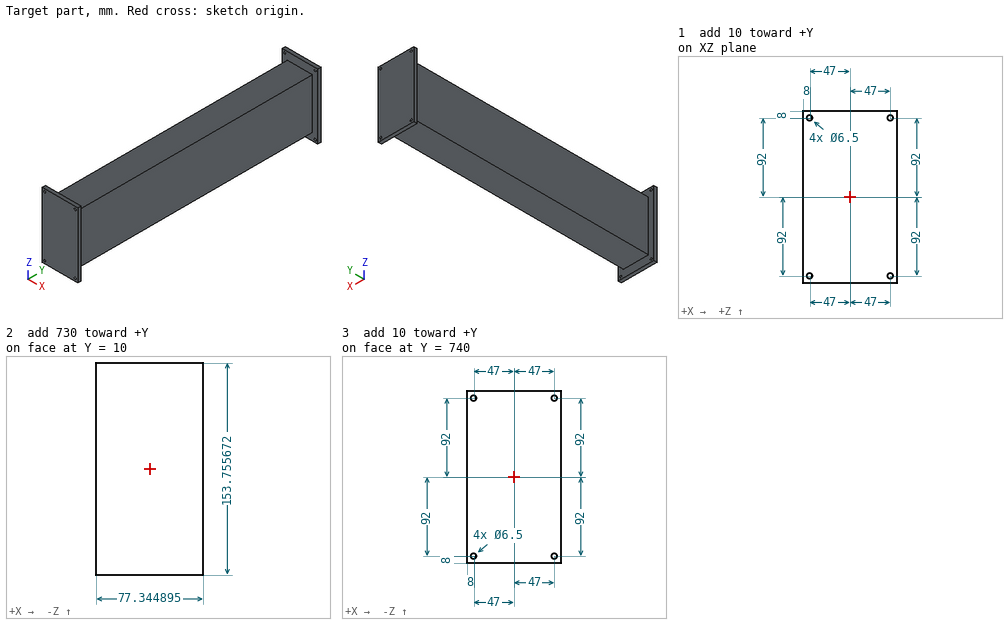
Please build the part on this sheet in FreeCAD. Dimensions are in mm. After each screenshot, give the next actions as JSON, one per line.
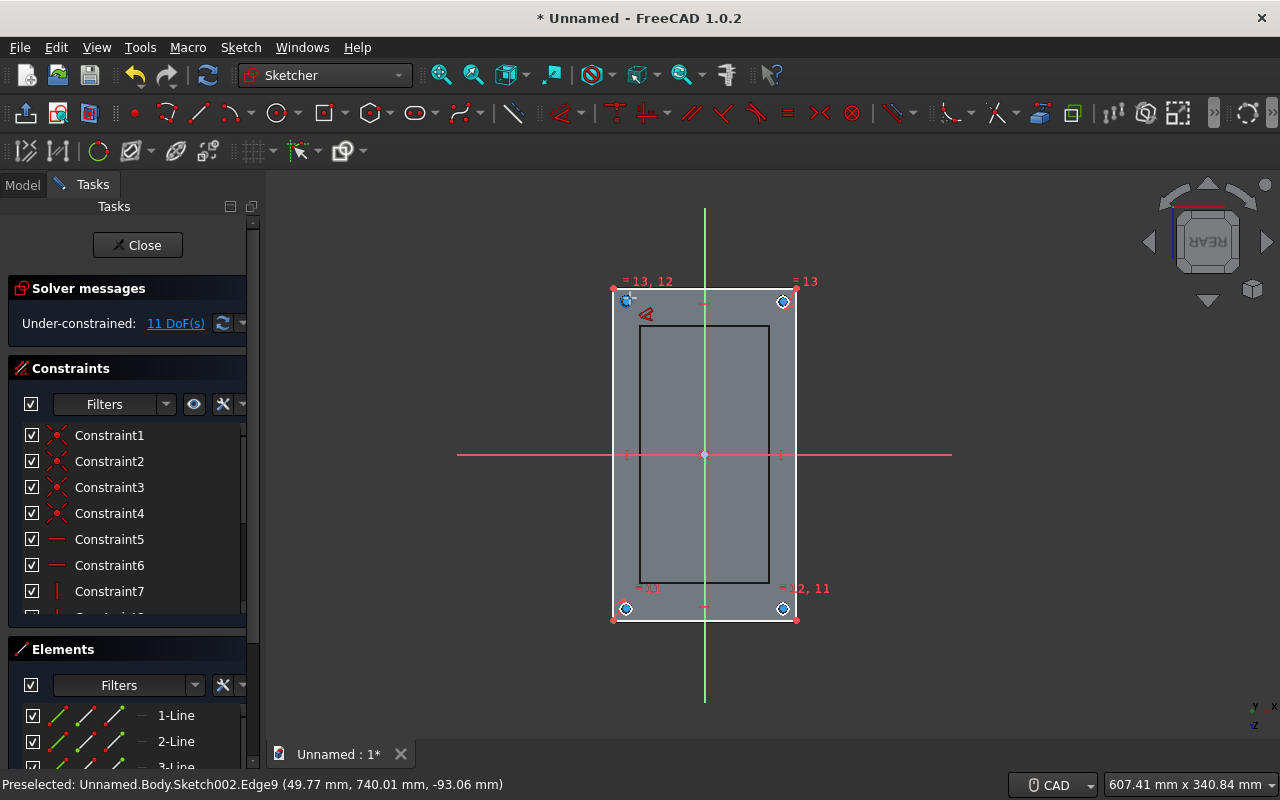
{"action": "scroll", "coordinate": [630, 605], "scroll_direction": "up", "scroll_amount": 7}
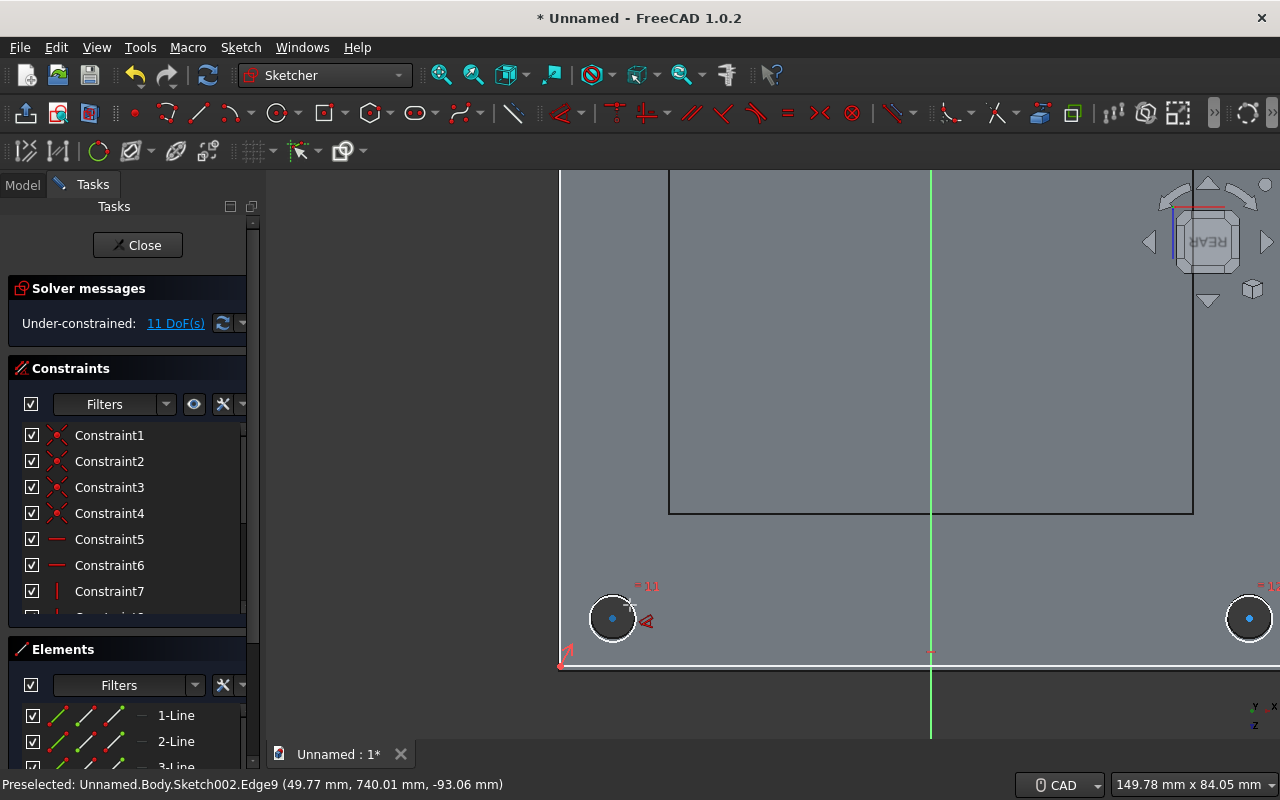
{"action": "left_click", "coordinate": [629, 603]}
{"action": "left_click", "coordinate": [652, 581]}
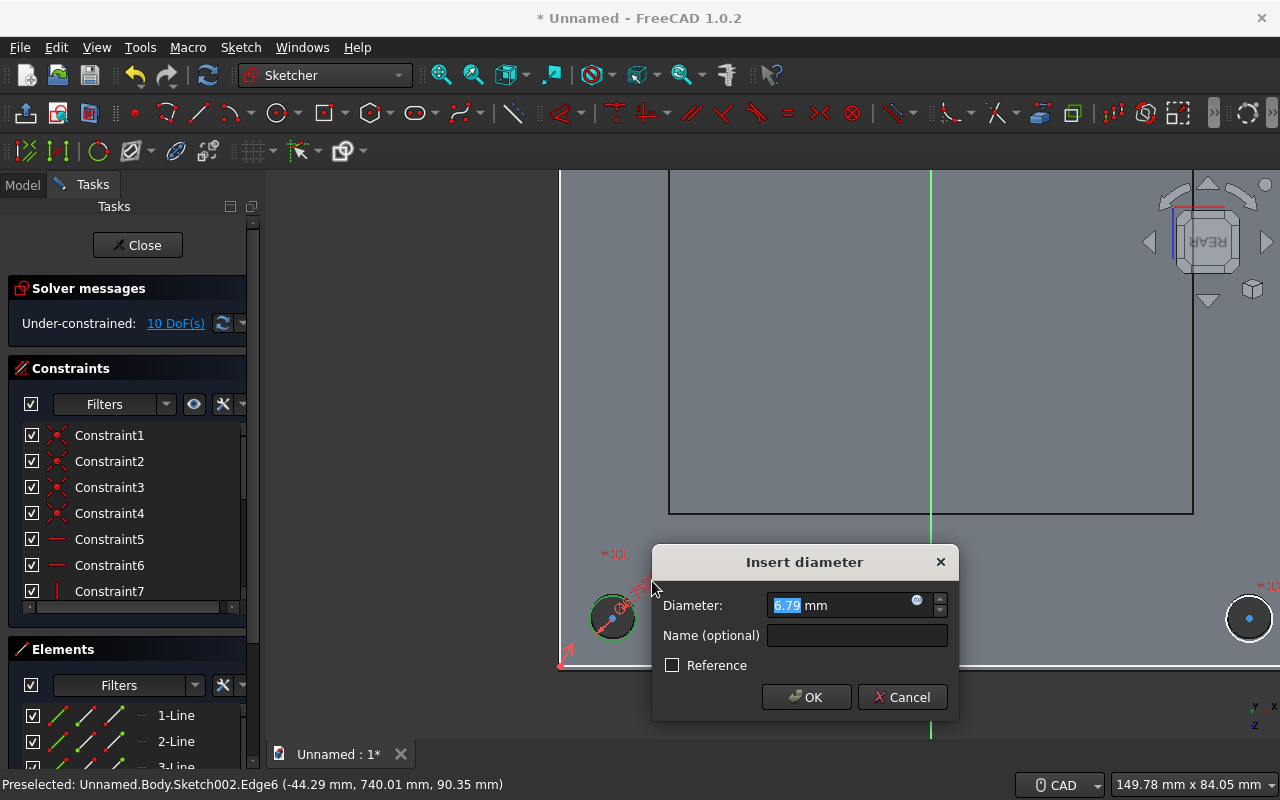
{"action": "type", "text": "6.5"}
{"action": "key", "text": "Return"}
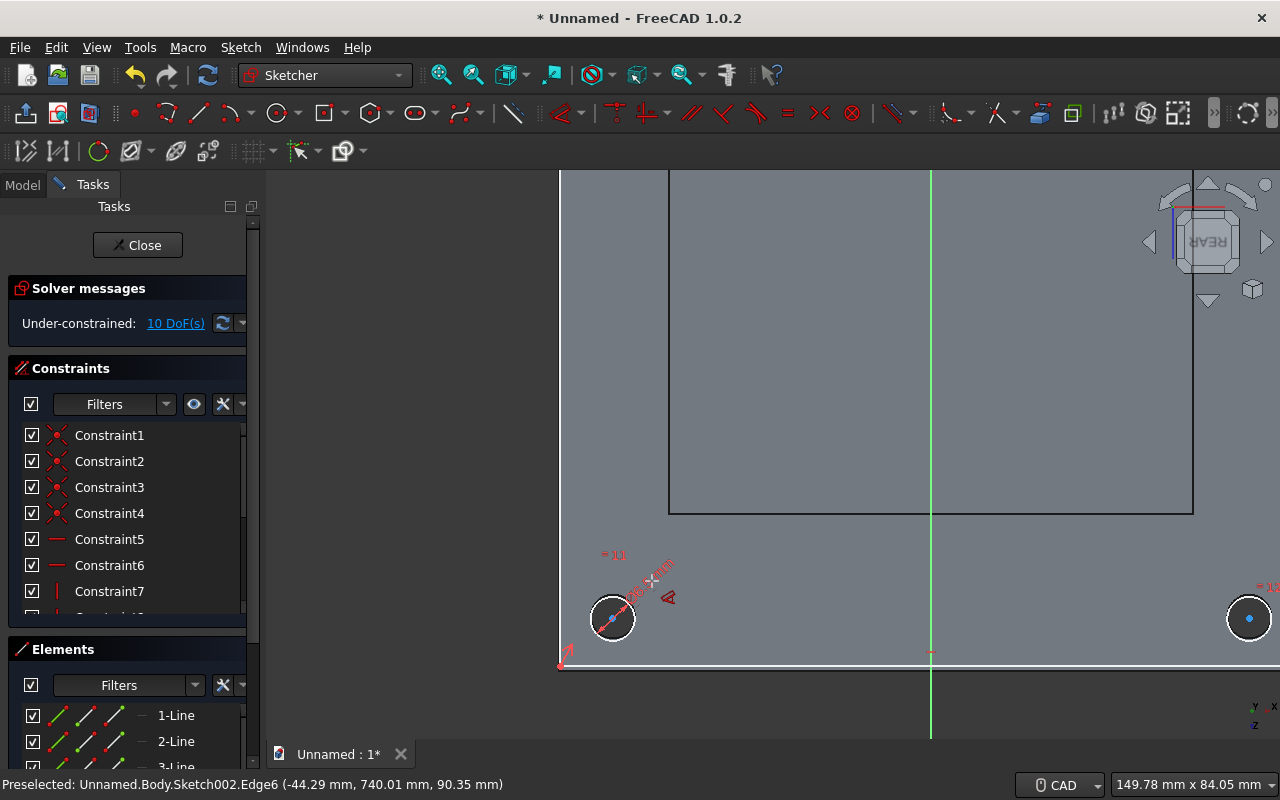
{"action": "scroll", "coordinate": [630, 605], "scroll_direction": "down", "scroll_amount": 7}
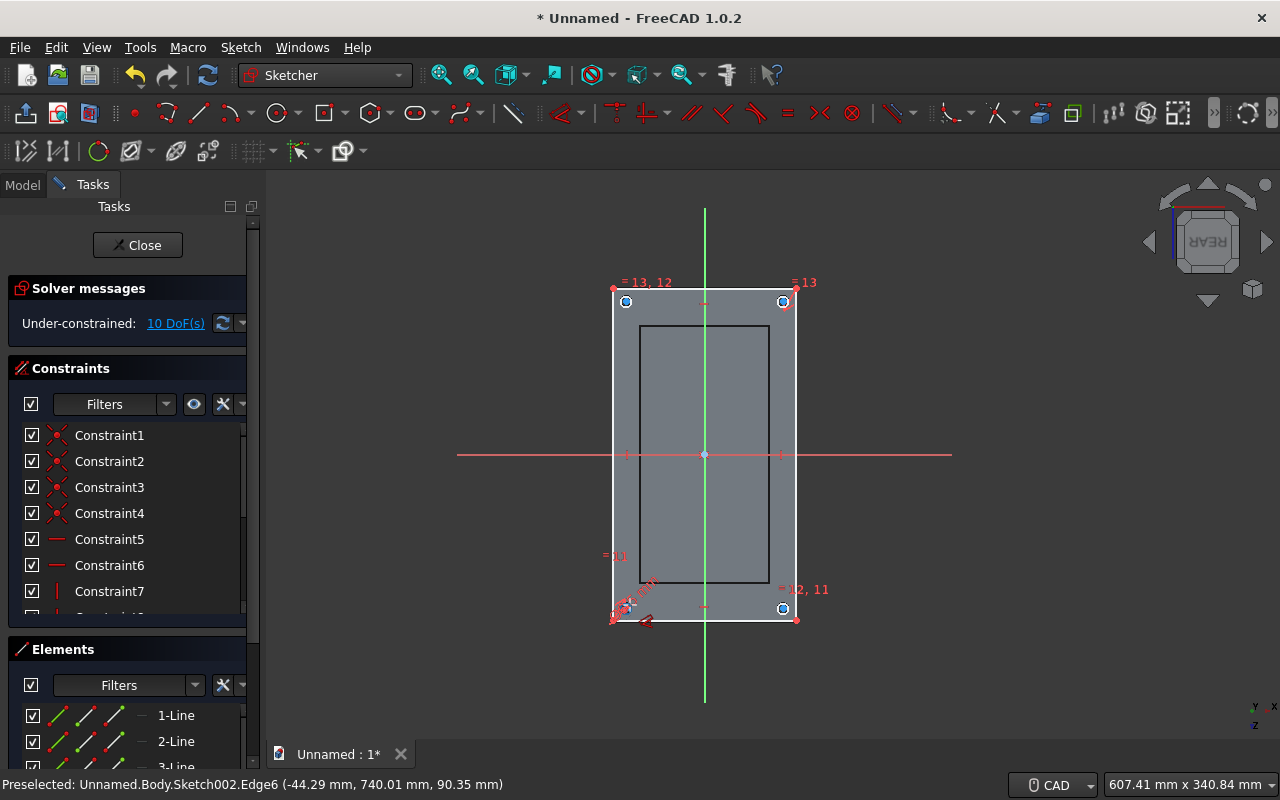
{"action": "left_click", "coordinate": [626, 609]}
{"action": "left_click", "coordinate": [665, 643]}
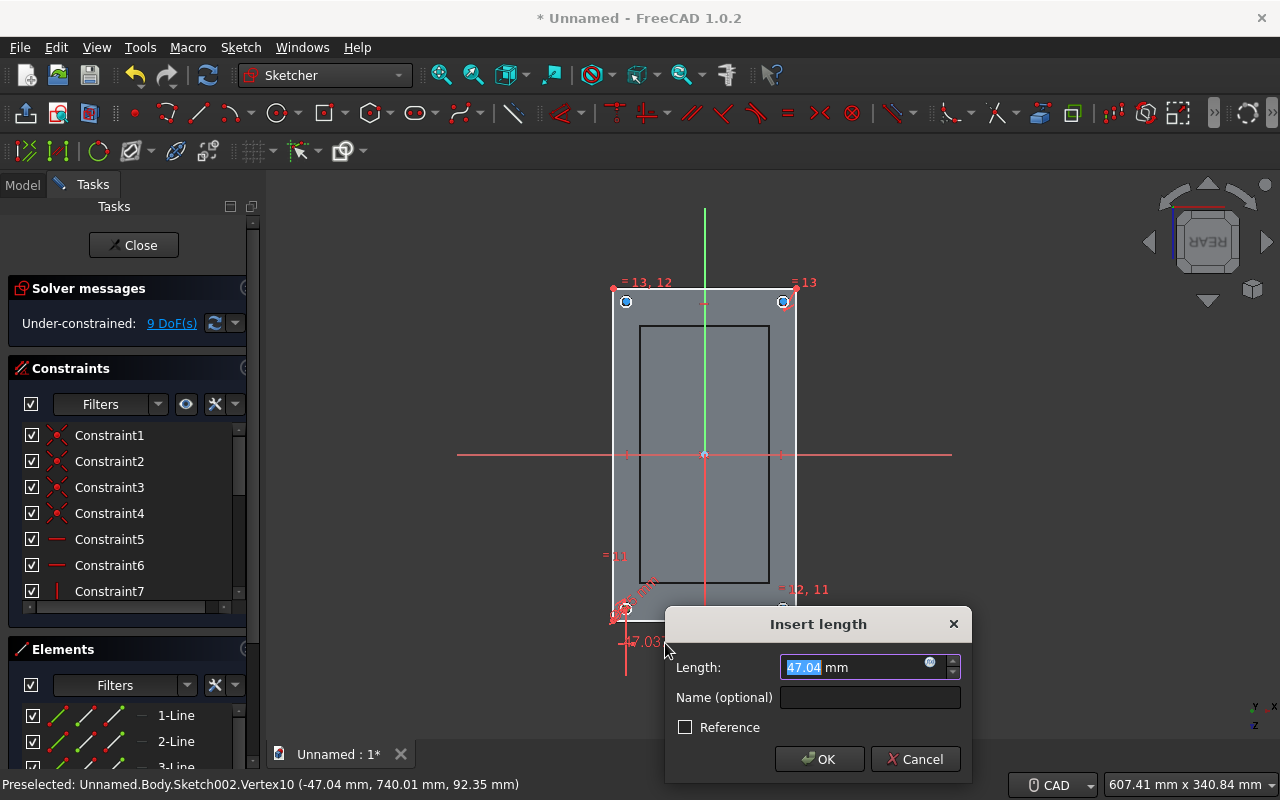
{"action": "type", "text": "47"}
{"action": "key", "text": "Return"}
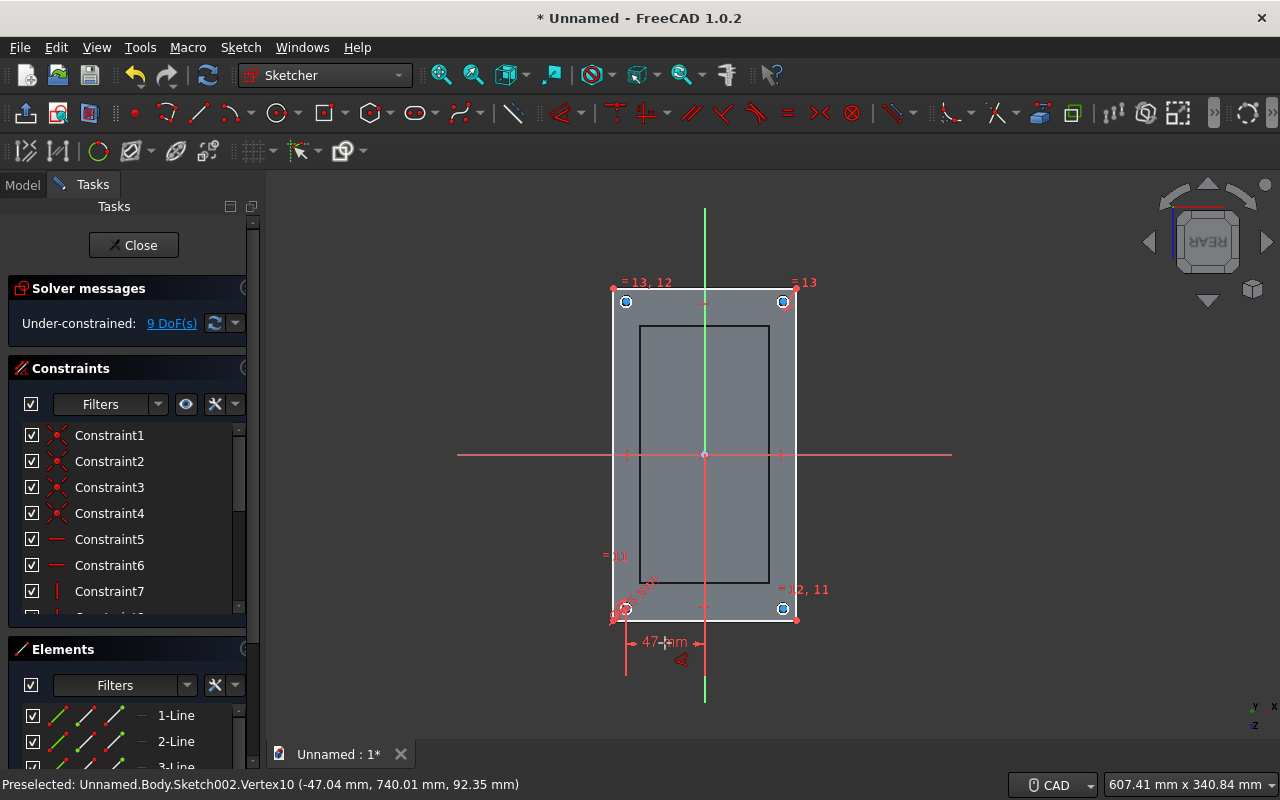
{"action": "left_click", "coordinate": [626, 609]}
{"action": "left_click", "coordinate": [592, 532]}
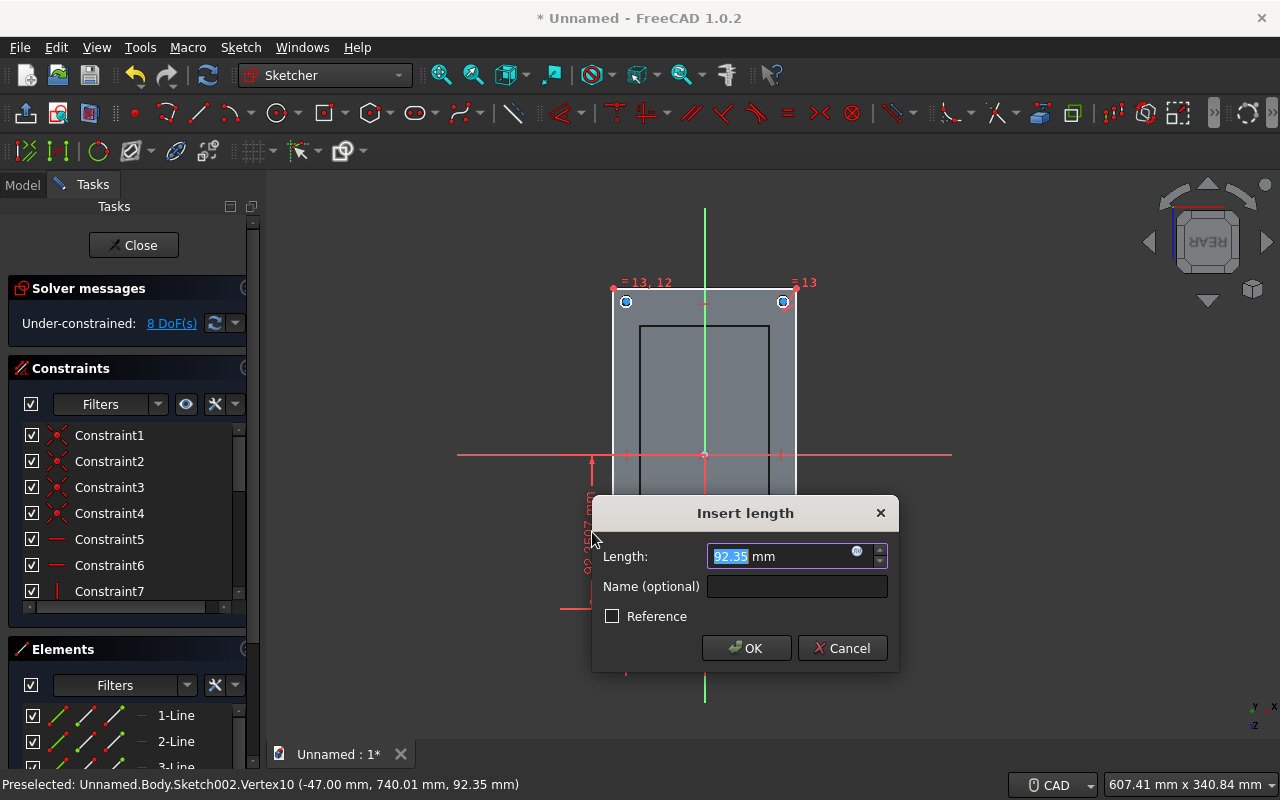
{"action": "type", "text": "92"}
{"action": "key", "text": "Return"}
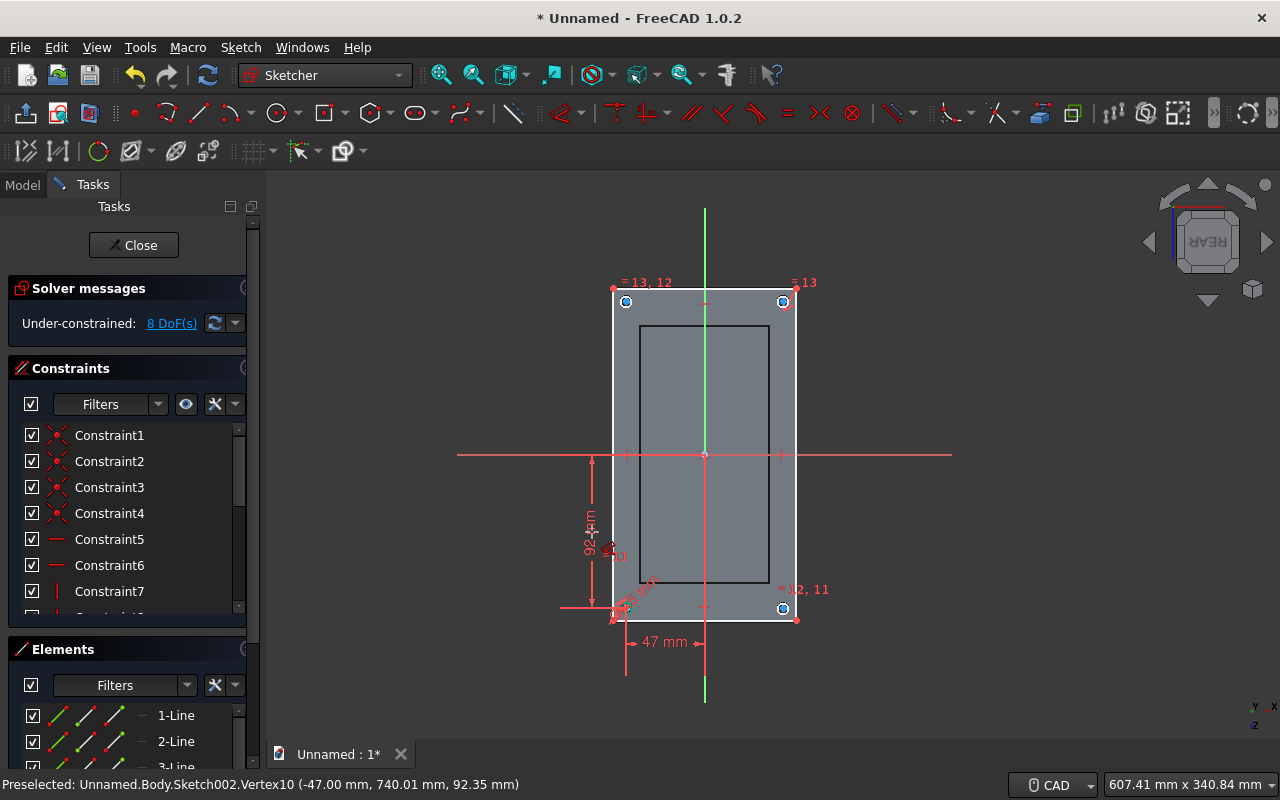
{"action": "left_click", "coordinate": [783, 609]}
{"action": "left_click", "coordinate": [744, 643]}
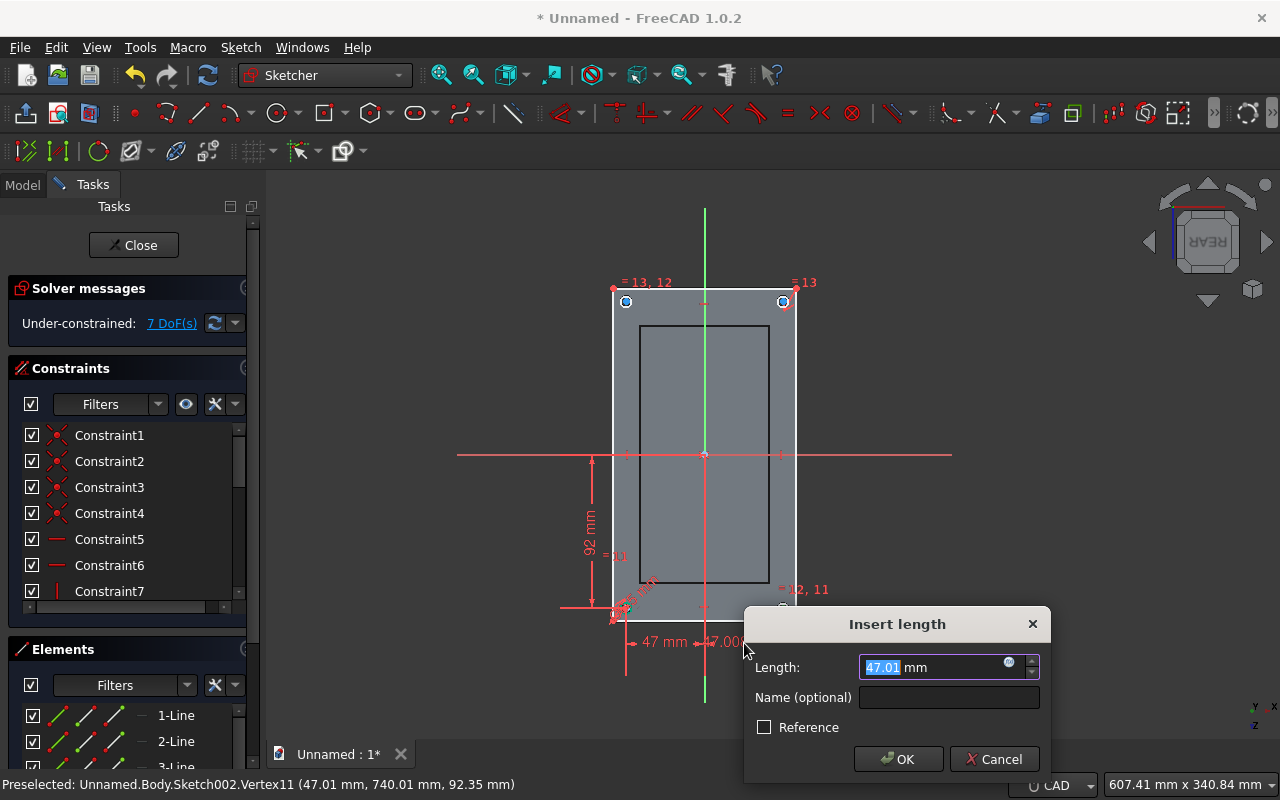
{"action": "type", "text": "47"}
{"action": "key", "text": "Return"}